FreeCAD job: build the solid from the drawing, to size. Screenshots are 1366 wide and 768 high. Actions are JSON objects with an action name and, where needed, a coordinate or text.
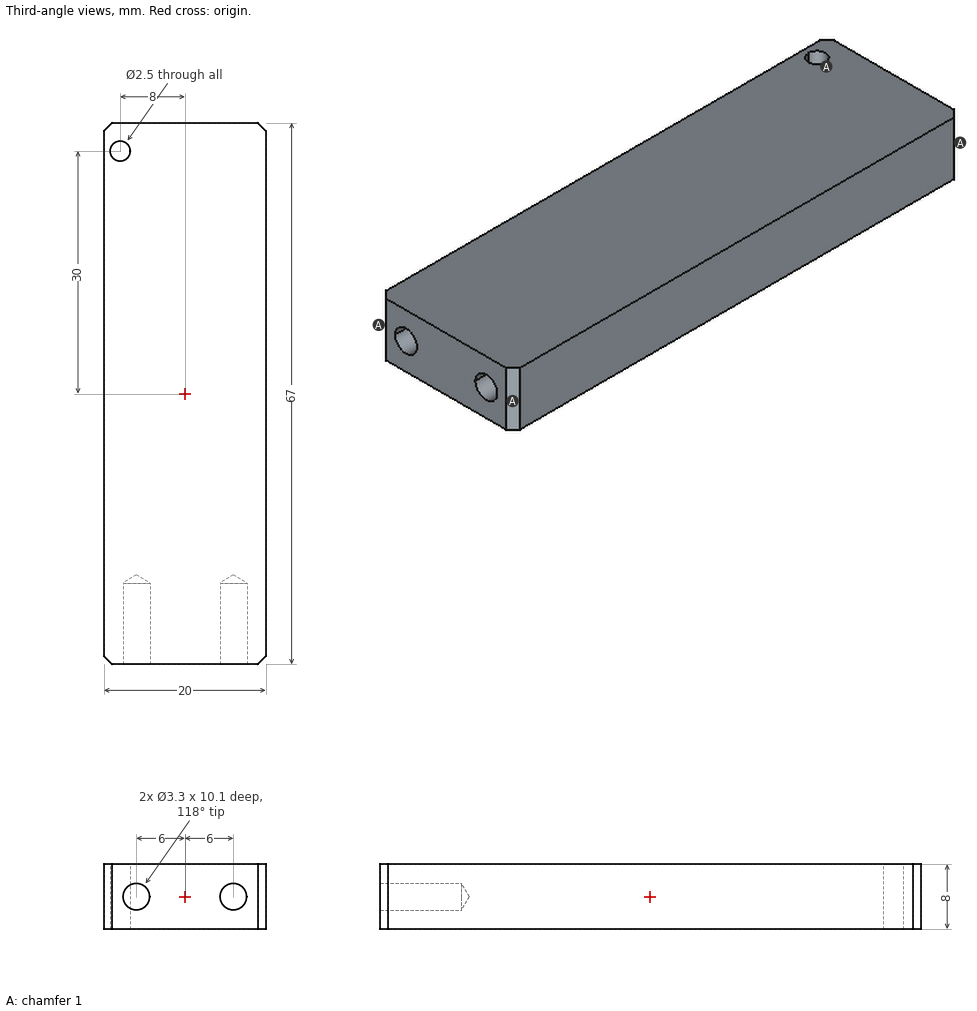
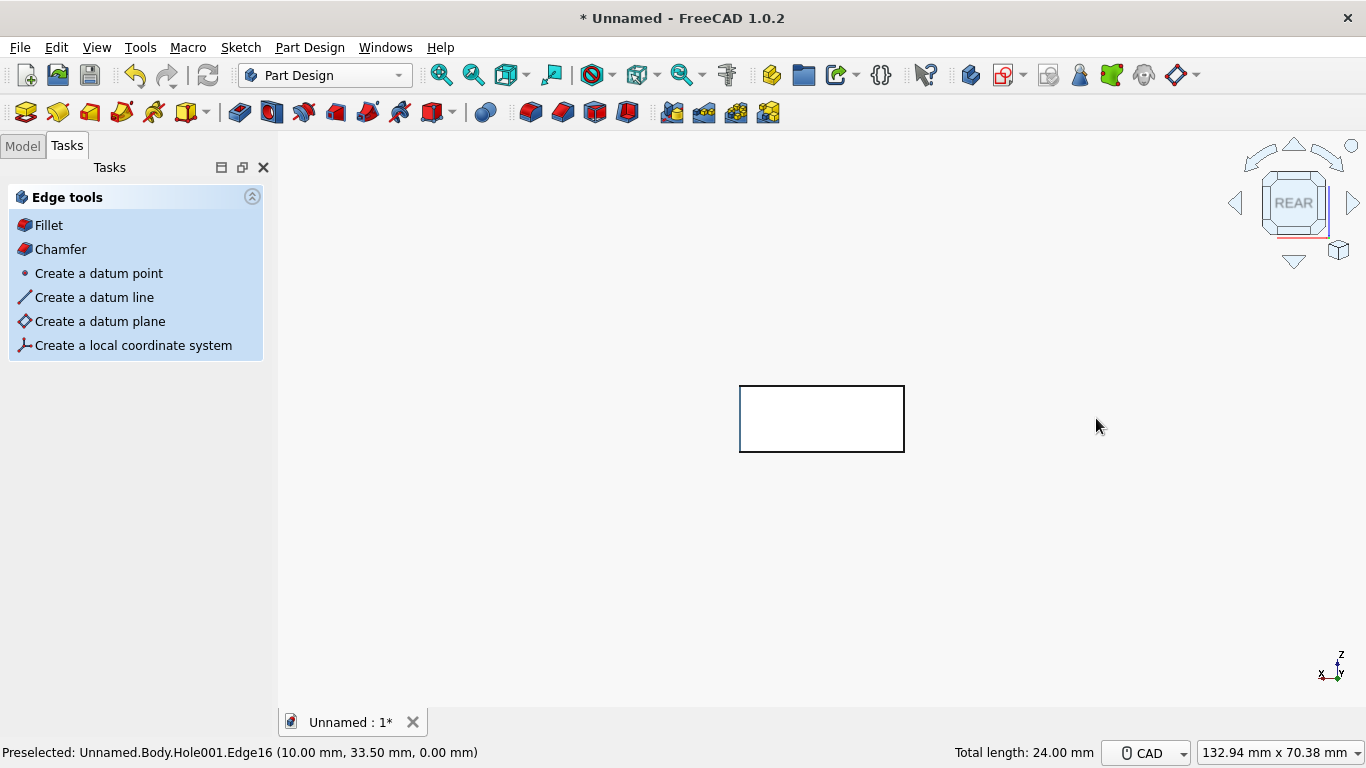
{"action": "key", "text": "v f"}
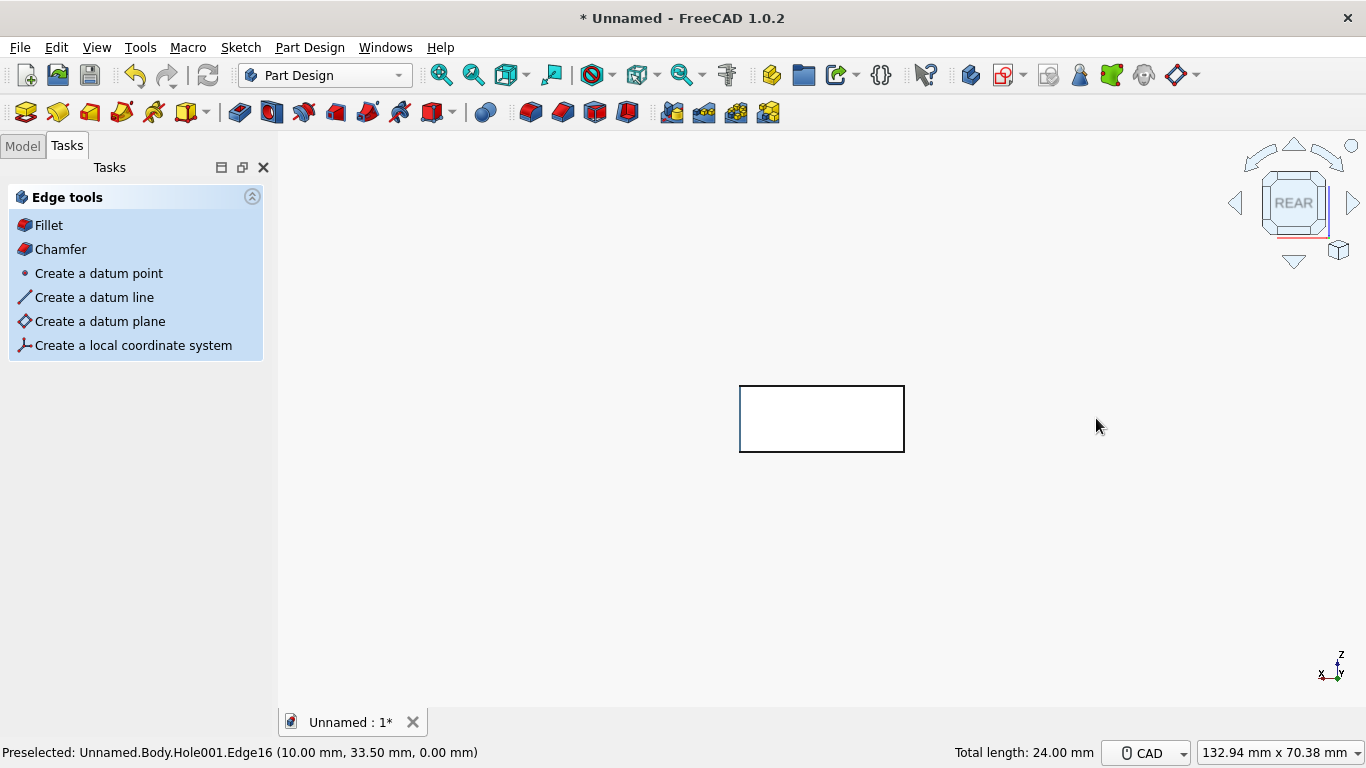
{"action": "left_click", "coordinate": [904, 418], "text": "ctrl"}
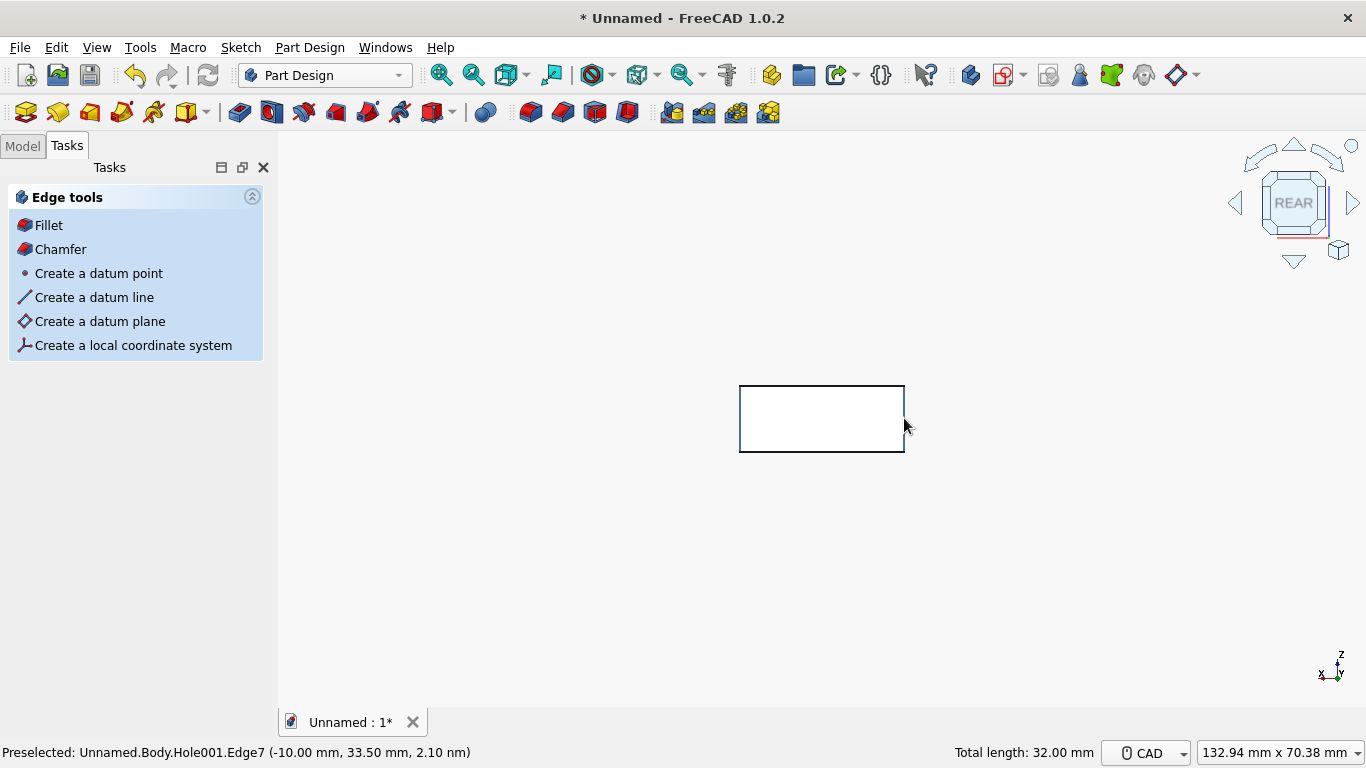
{"action": "left_click", "coordinate": [564, 112]}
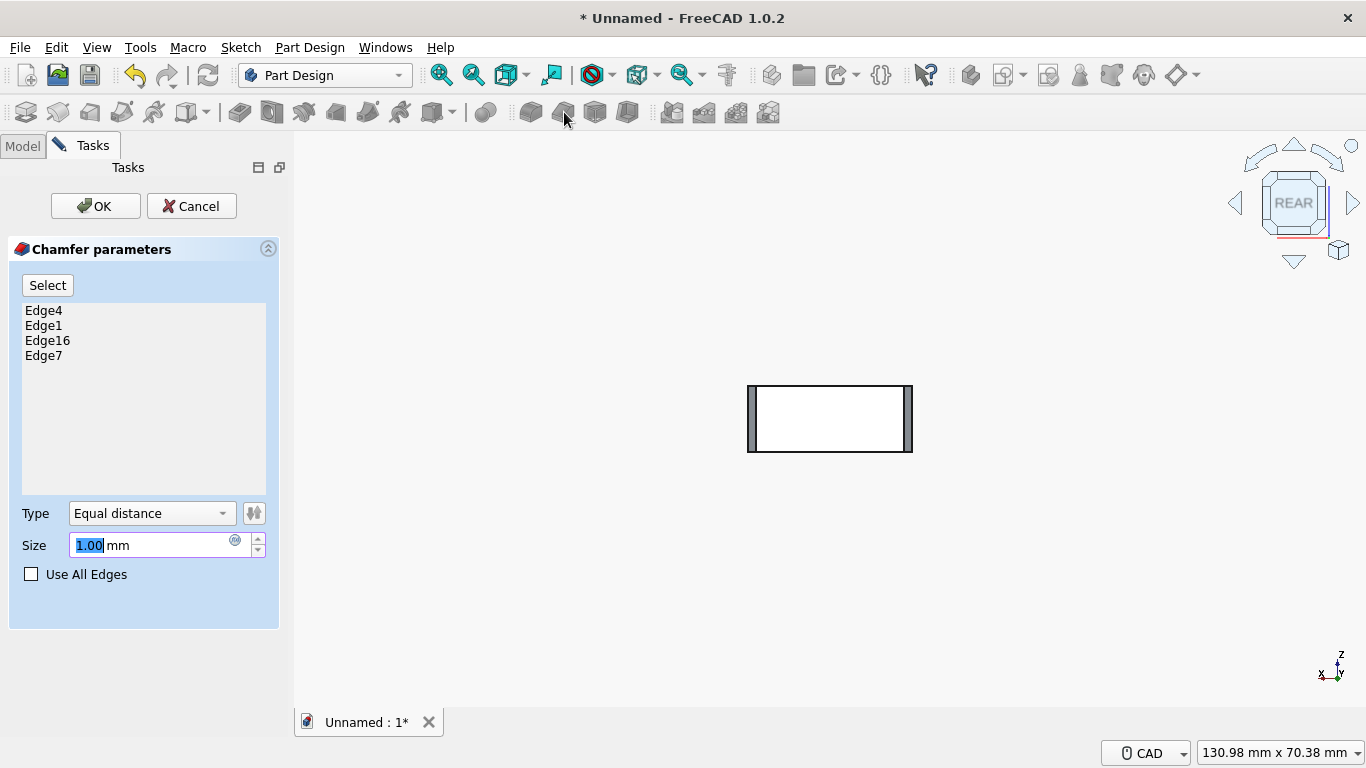
{"action": "type", "text": "1"}
{"action": "key", "text": "Tab"}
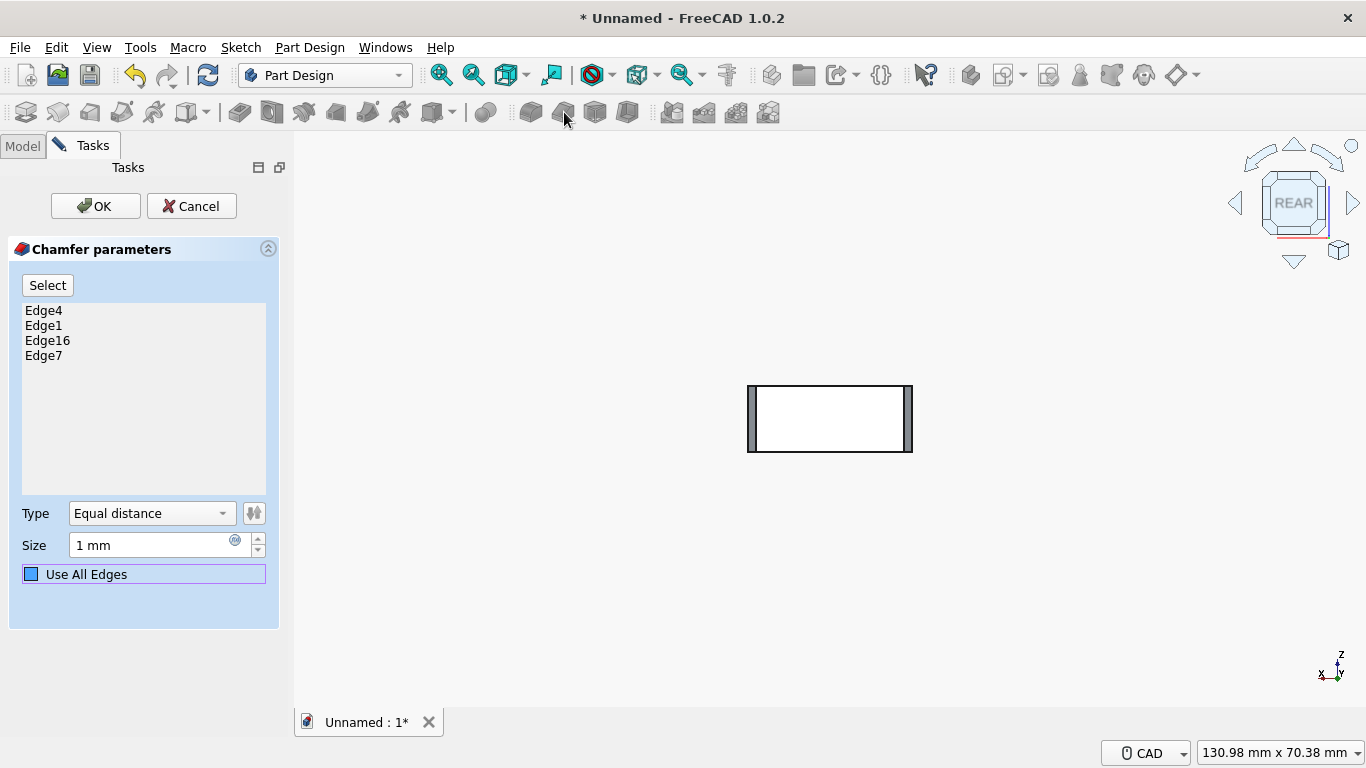
{"action": "left_click", "coordinate": [96, 206]}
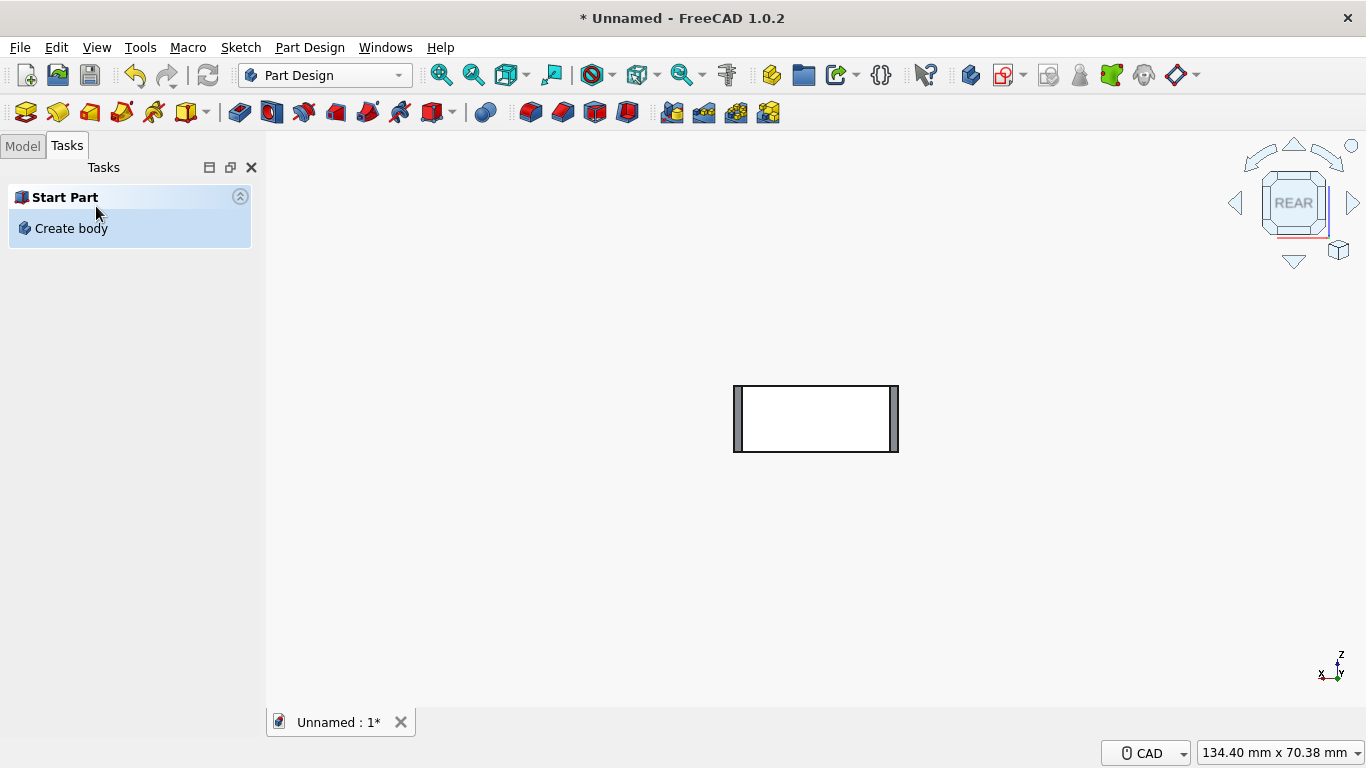
{"action": "key", "text": "0"}